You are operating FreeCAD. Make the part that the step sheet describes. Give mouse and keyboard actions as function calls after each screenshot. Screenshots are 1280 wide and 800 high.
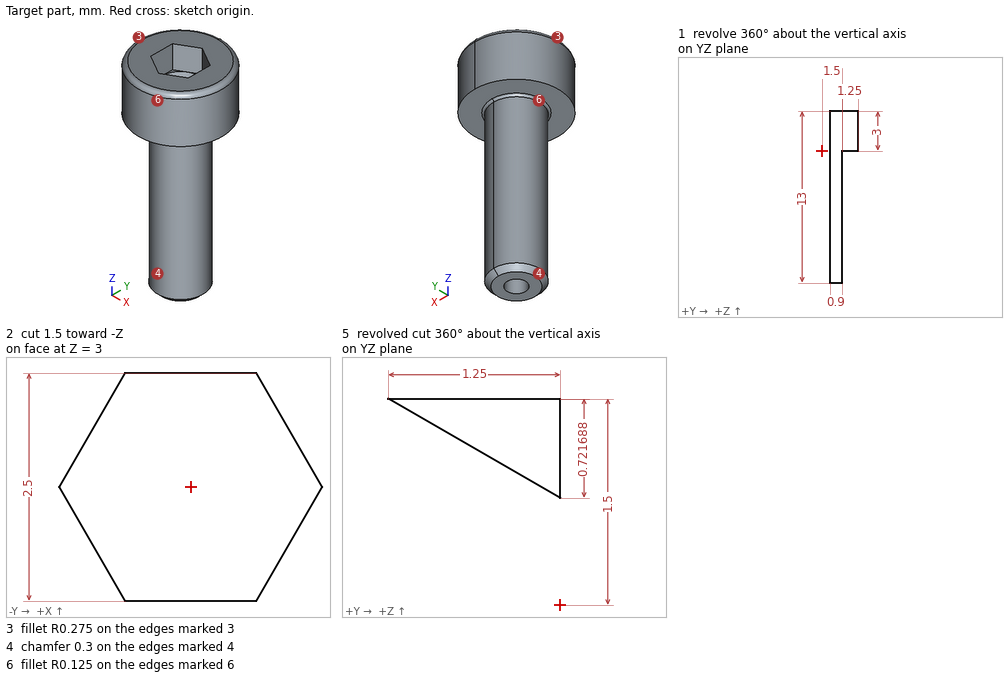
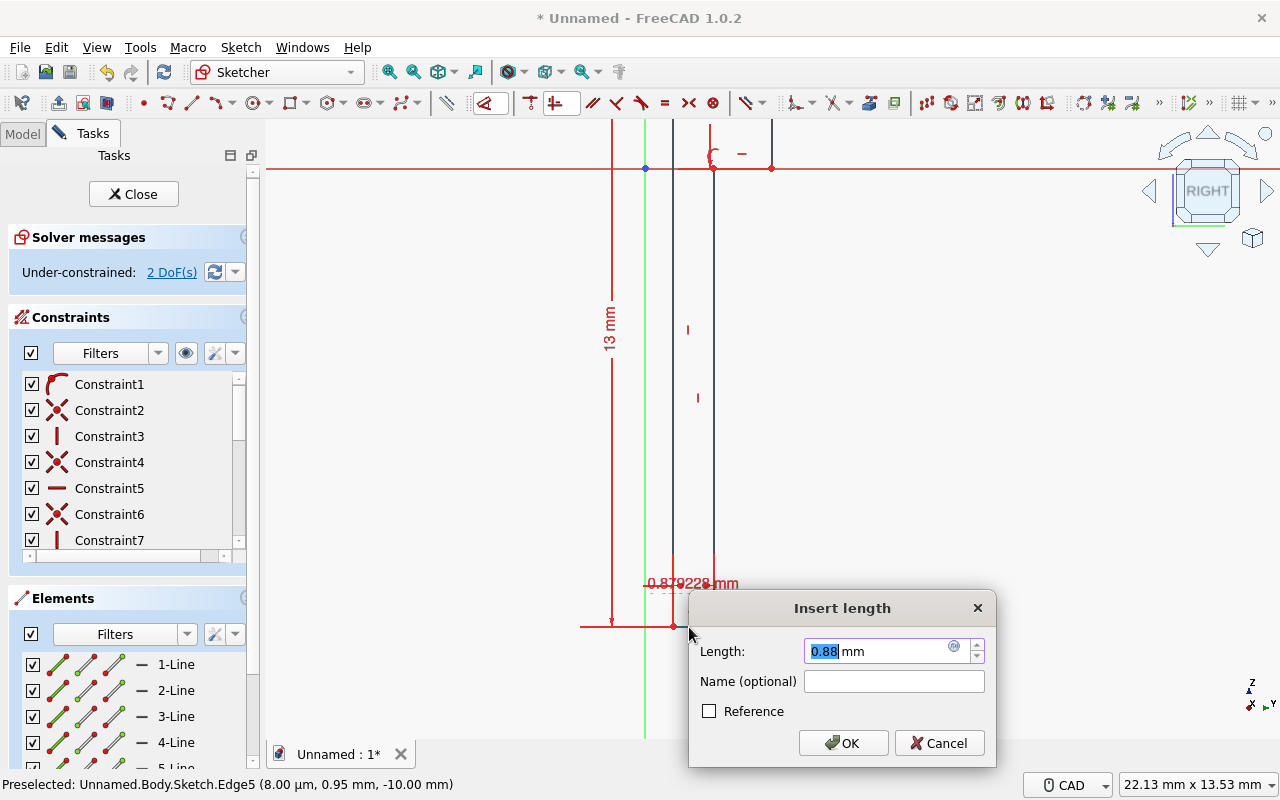
text(0.9)
key(Return)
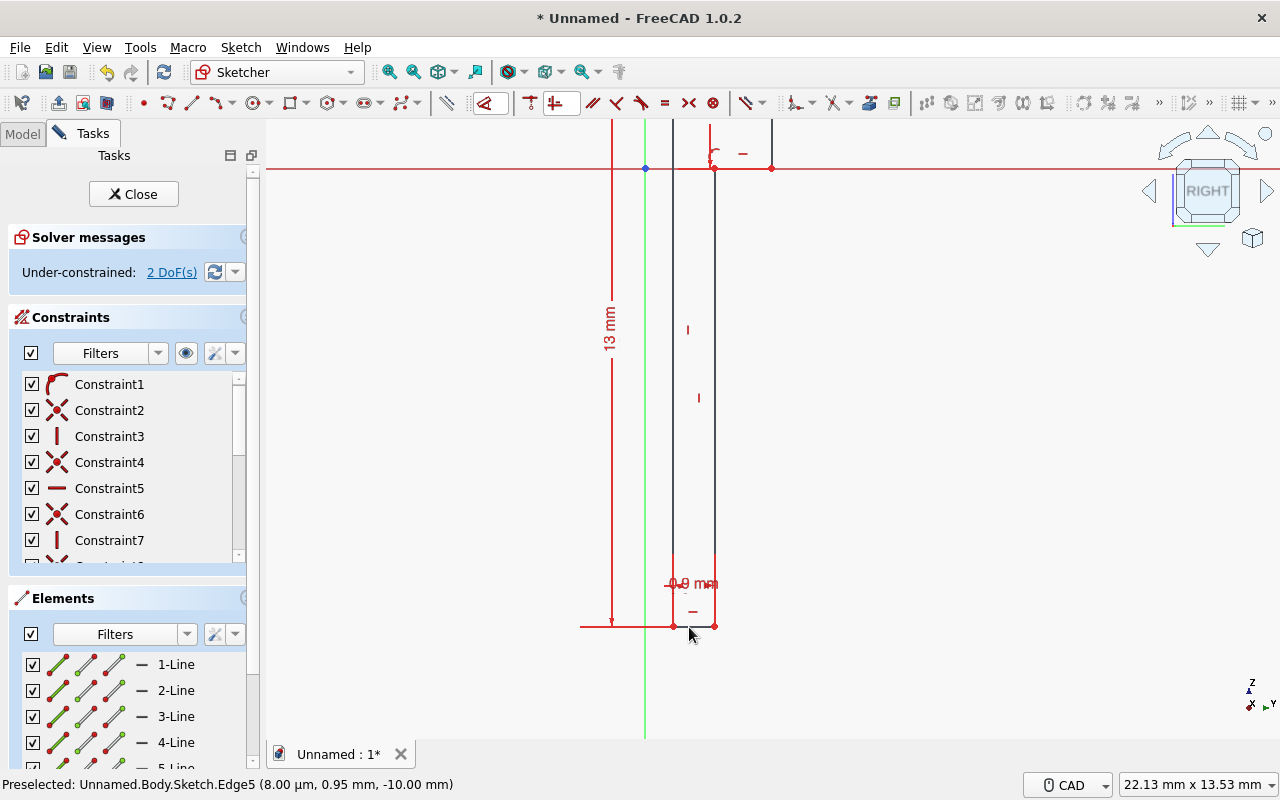
click(732, 169)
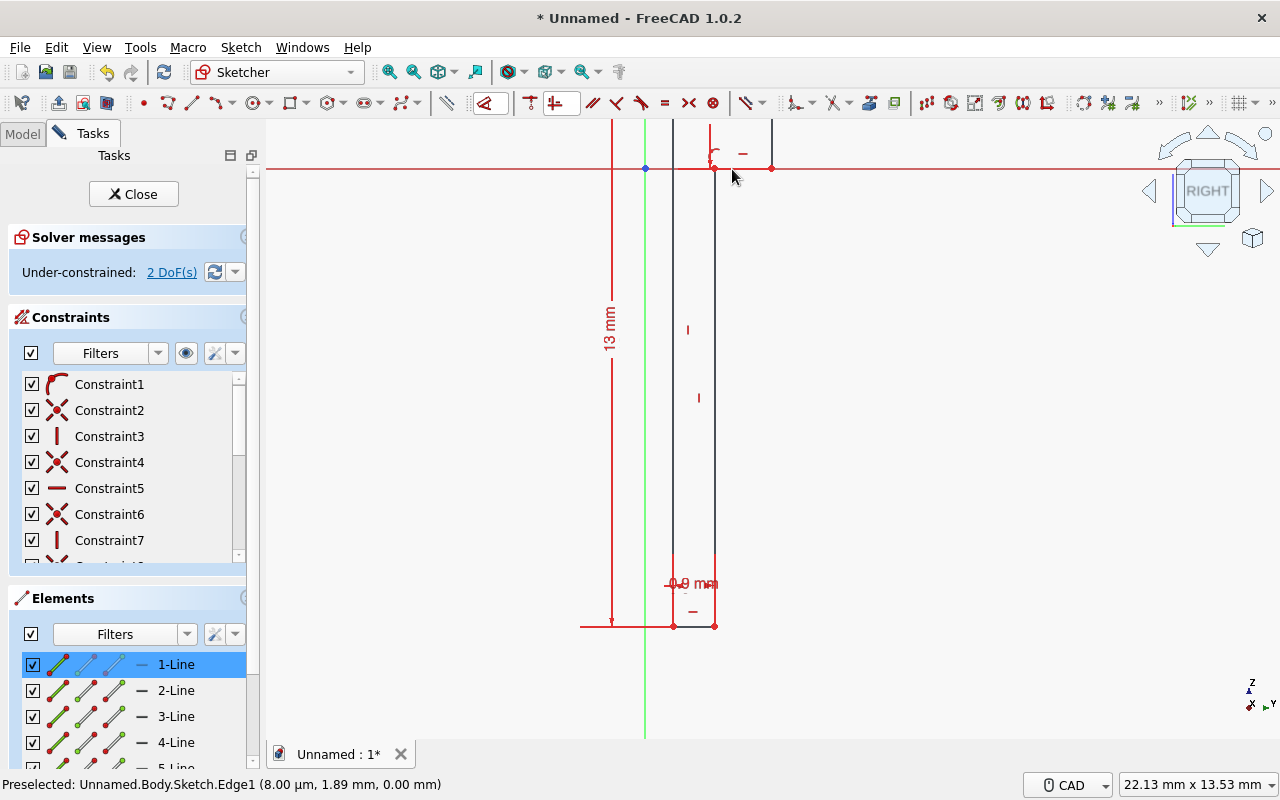
click(502, 104)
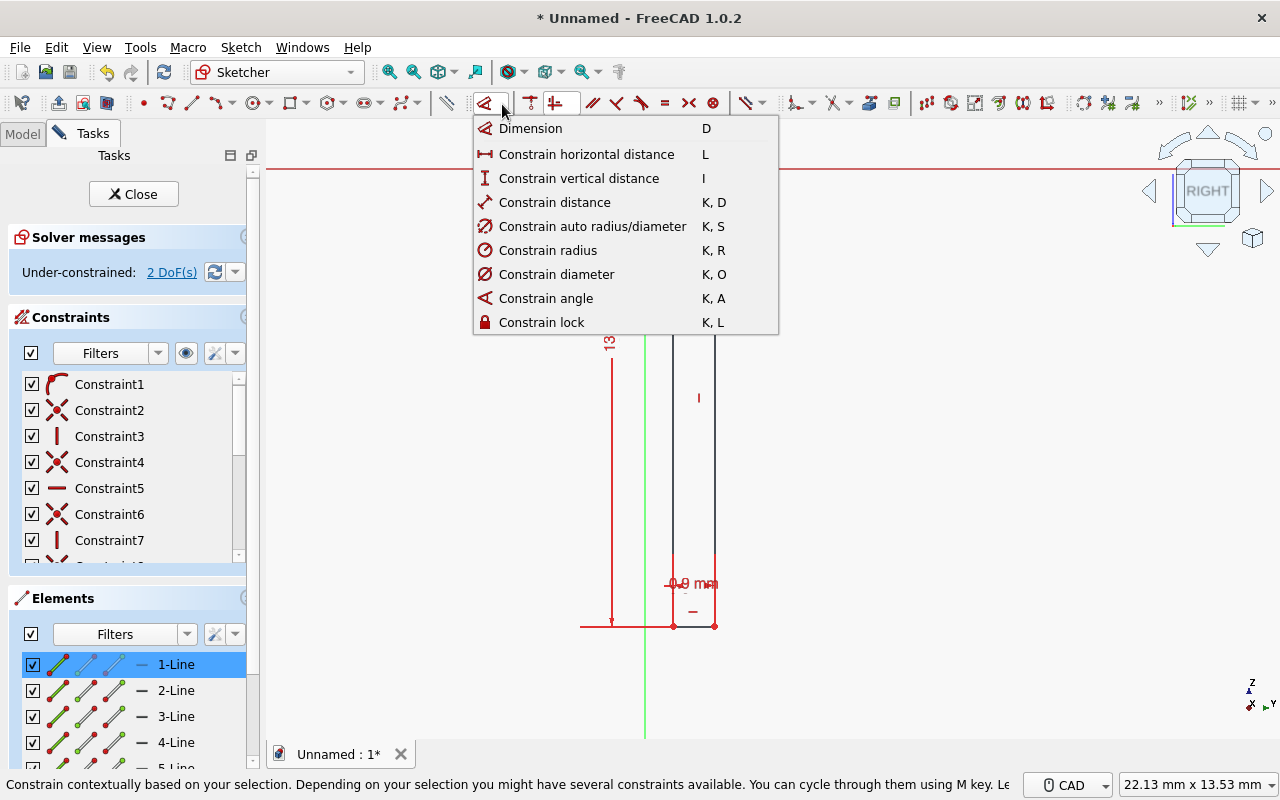
click(626, 154)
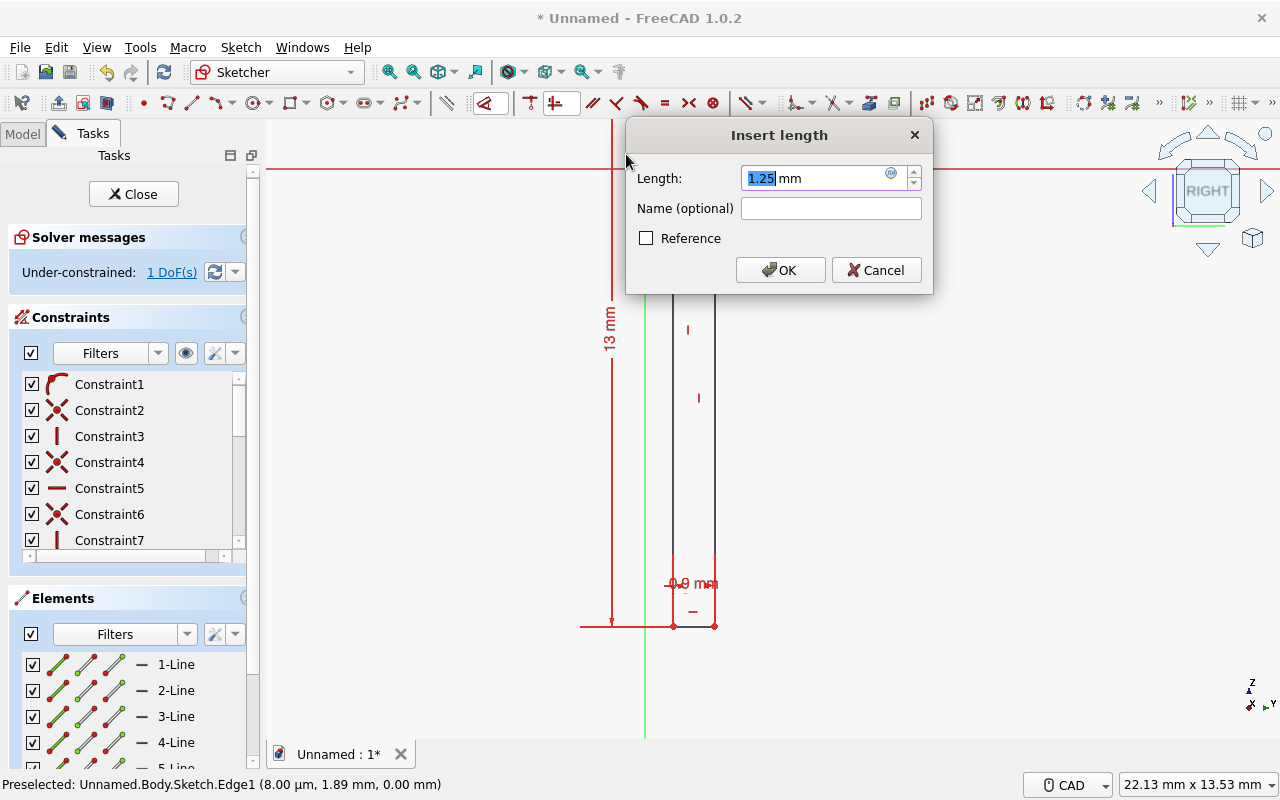
text(1.25)
key(Return)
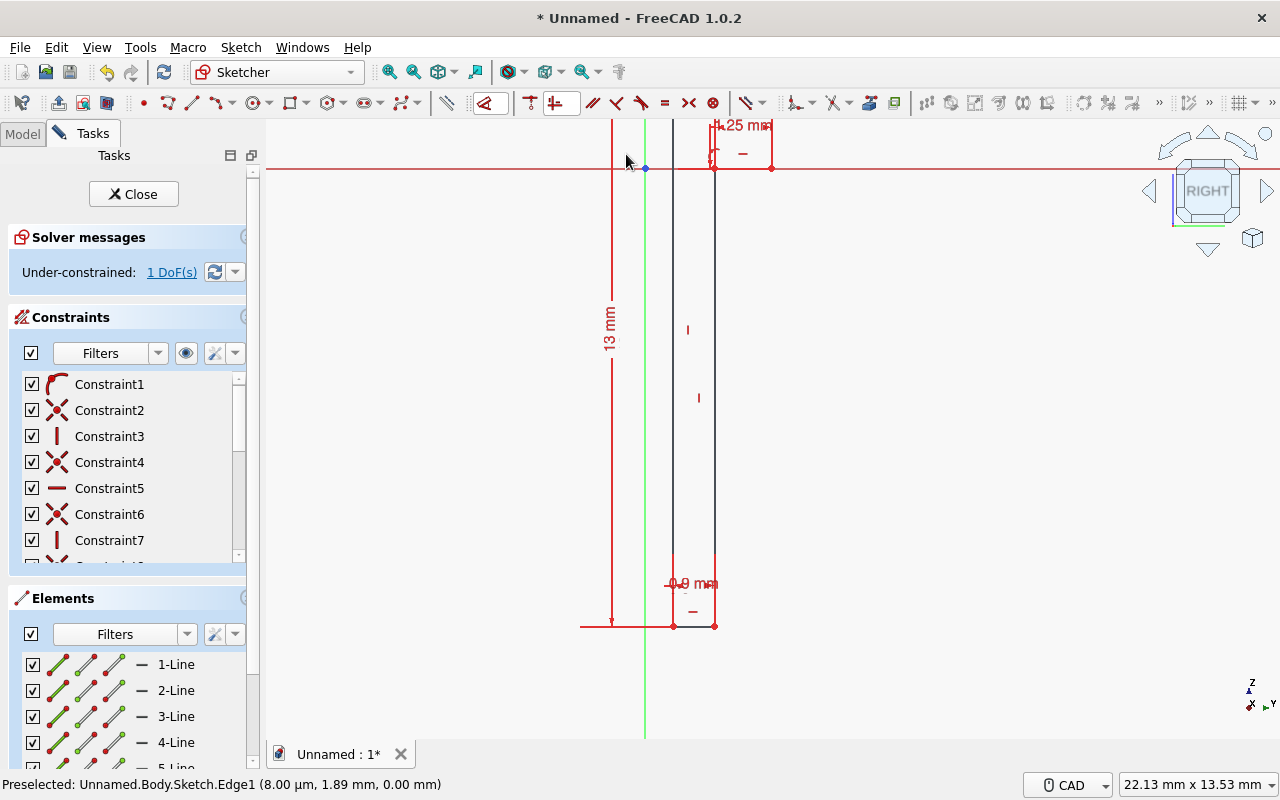
click(715, 169)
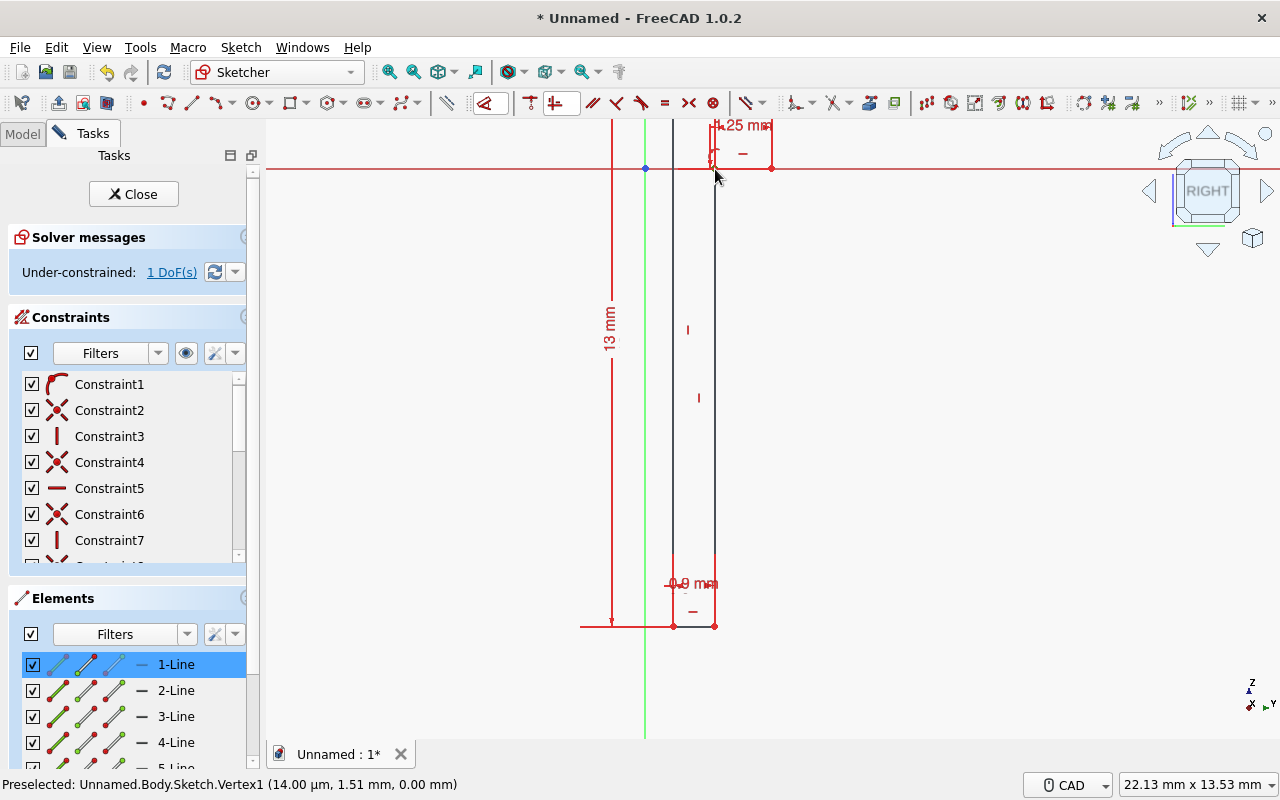
click(502, 104)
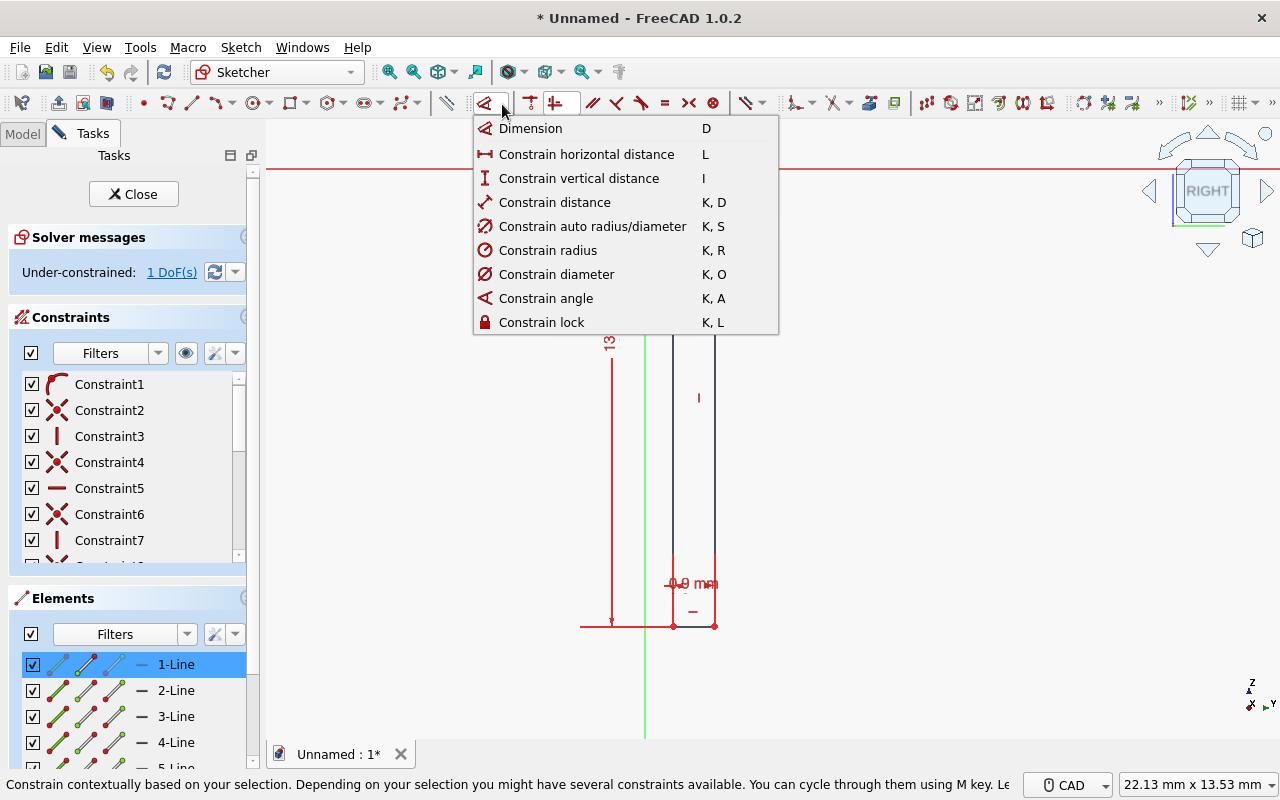
click(626, 154)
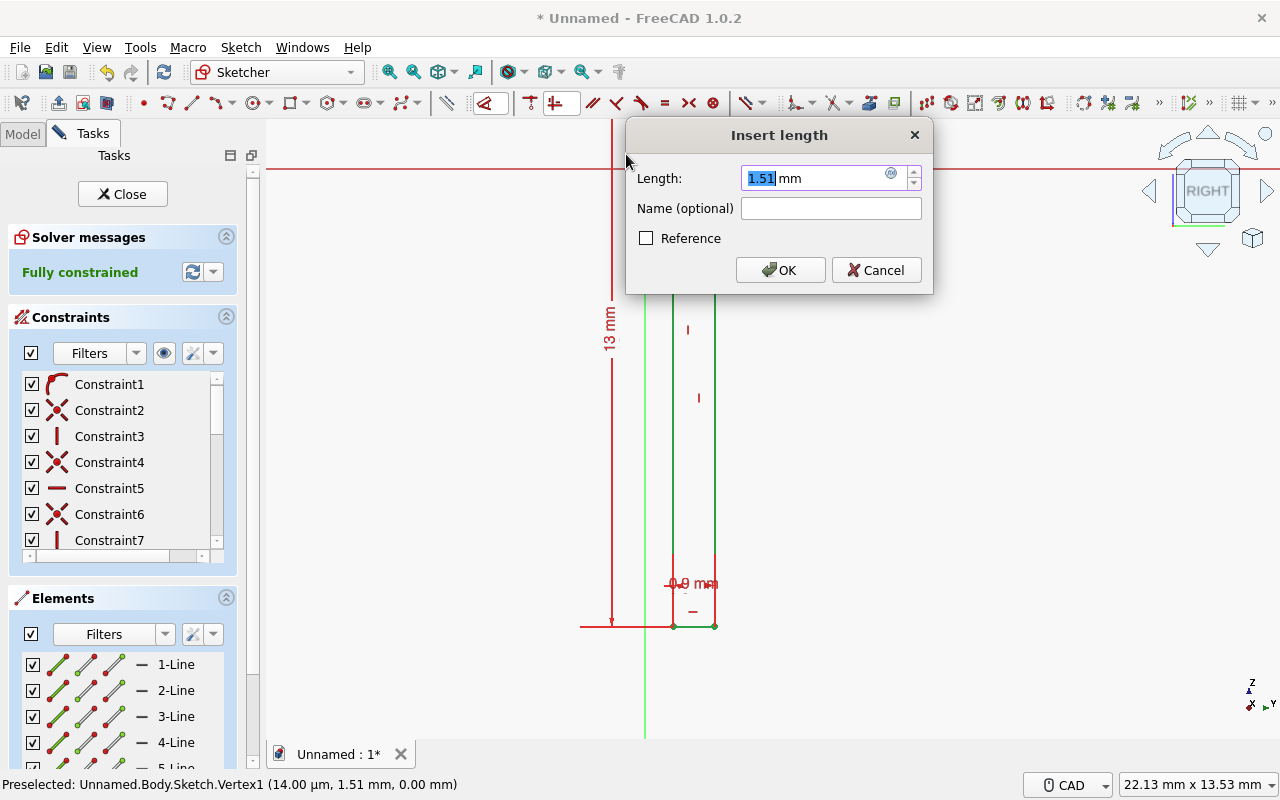
text(1.5)
key(Return)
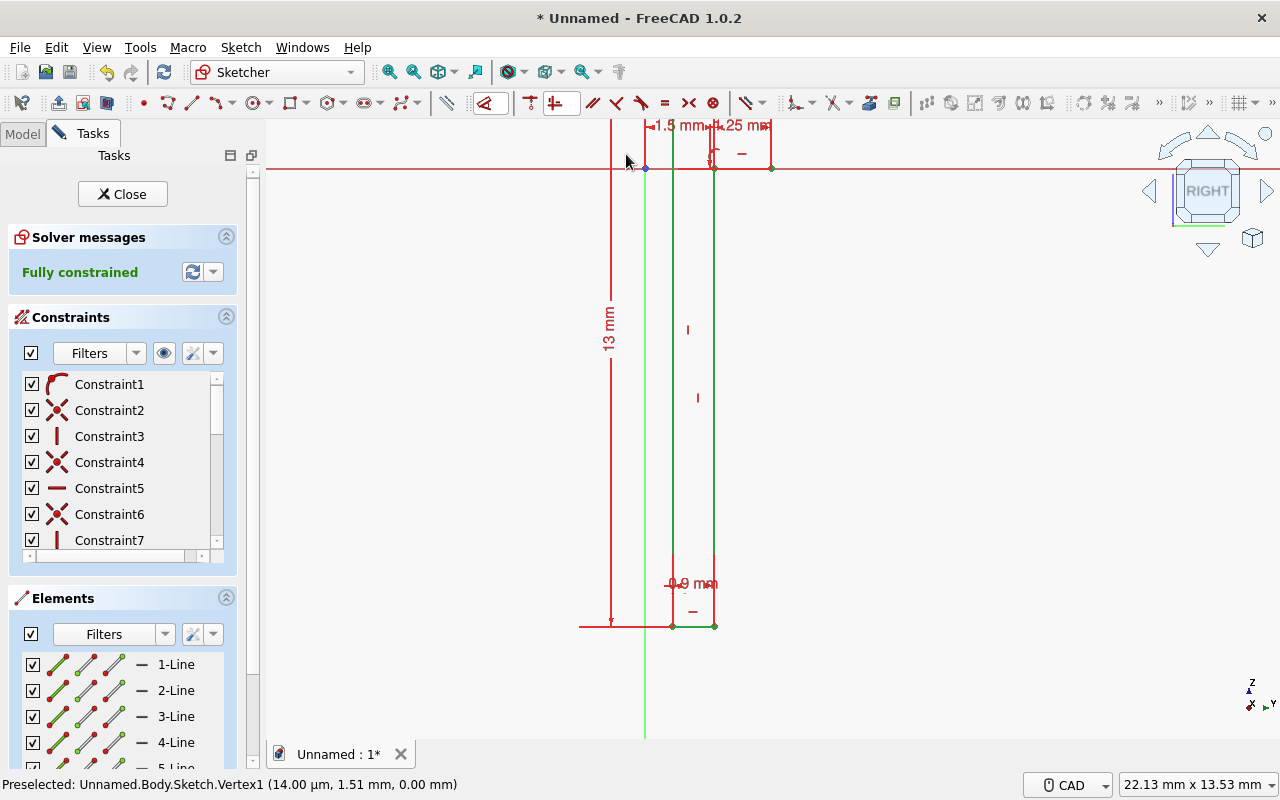
click(123, 194)